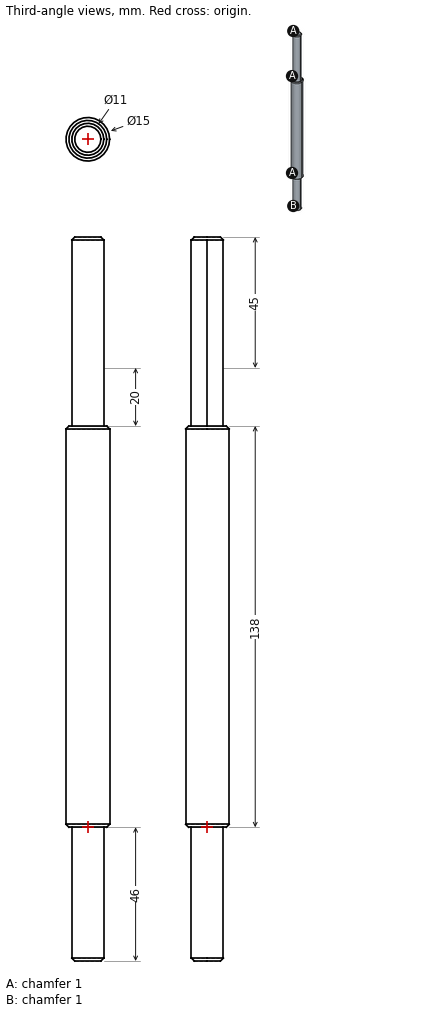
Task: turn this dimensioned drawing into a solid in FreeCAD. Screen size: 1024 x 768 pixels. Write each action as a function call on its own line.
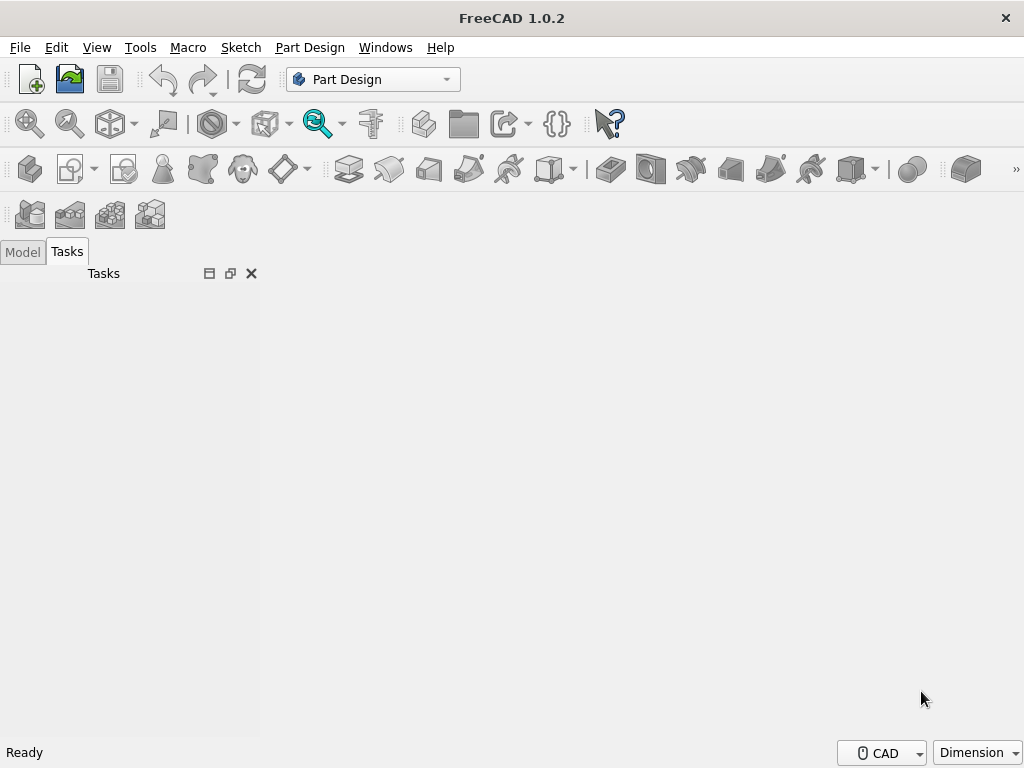
click(424, 170)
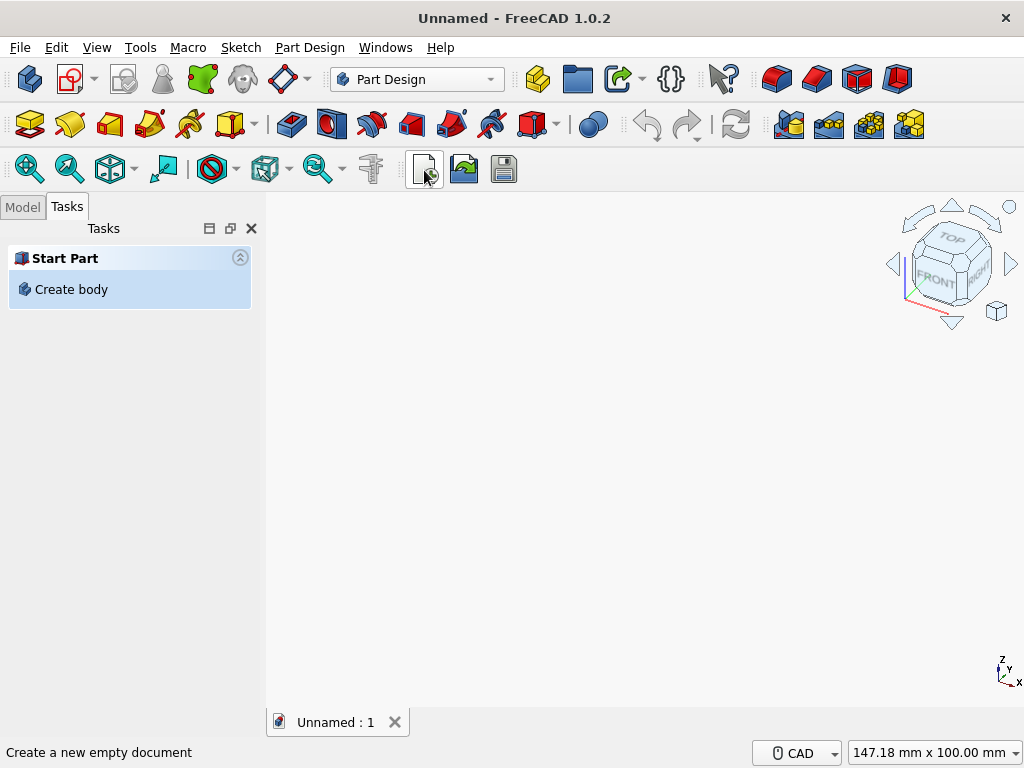
click(70, 80)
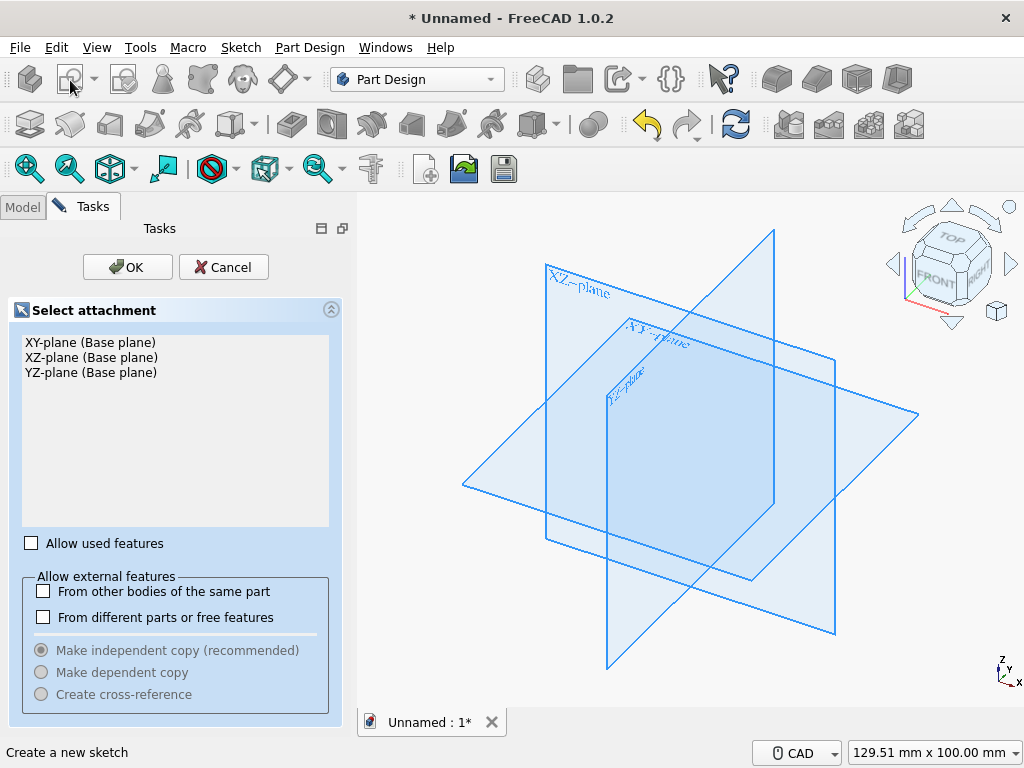
click(82, 342)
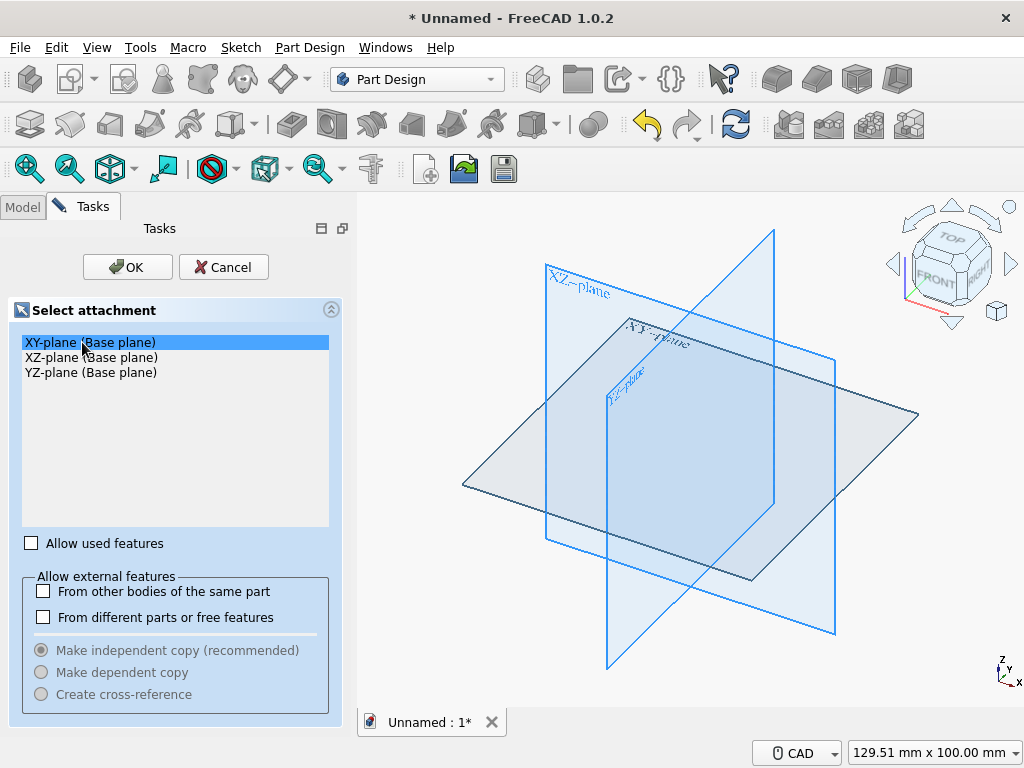
click(128, 267)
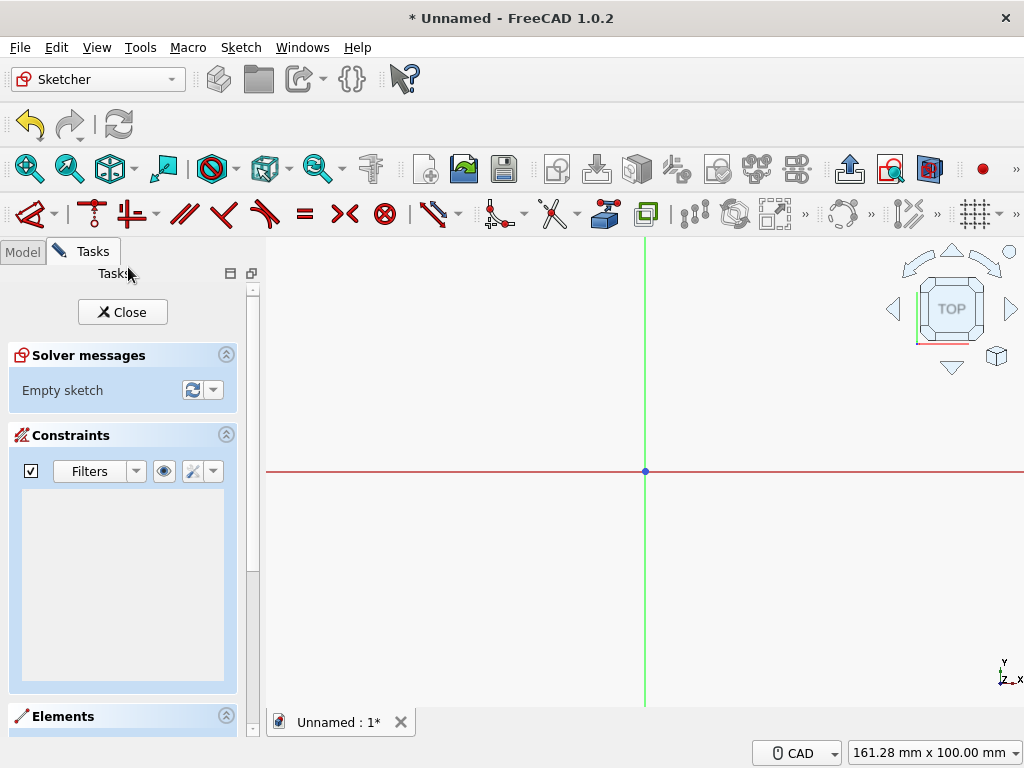
scroll(667, 472, up, 7)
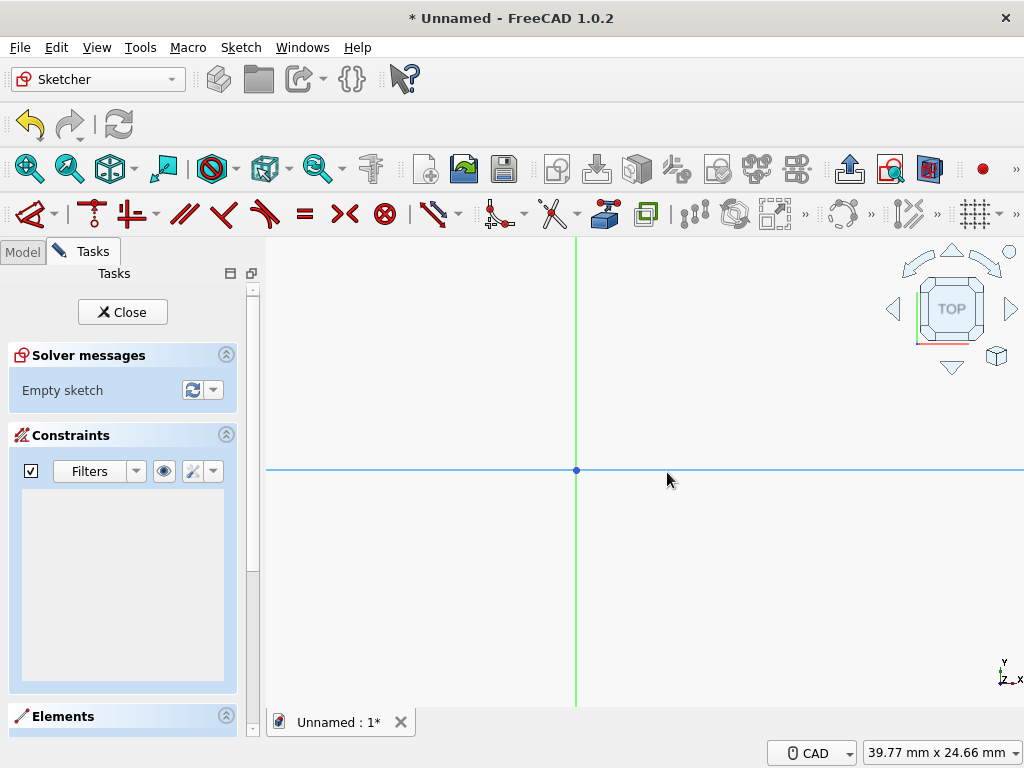
key(g)
key(c)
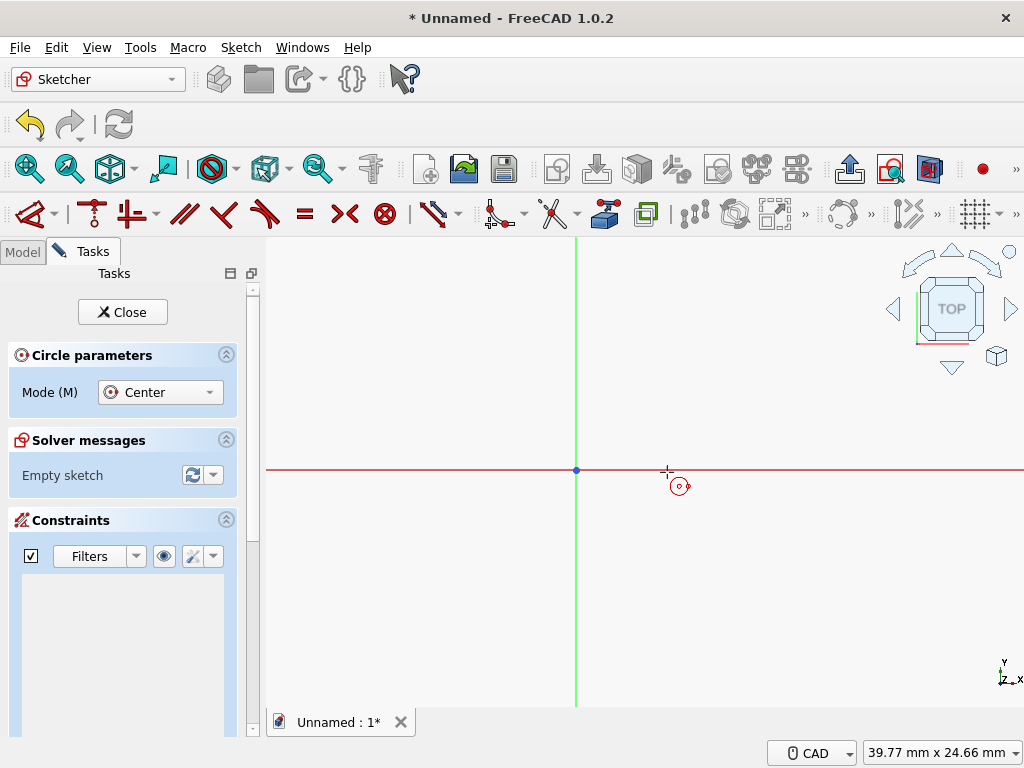
click(576, 470)
click(677, 369)
key(Escape)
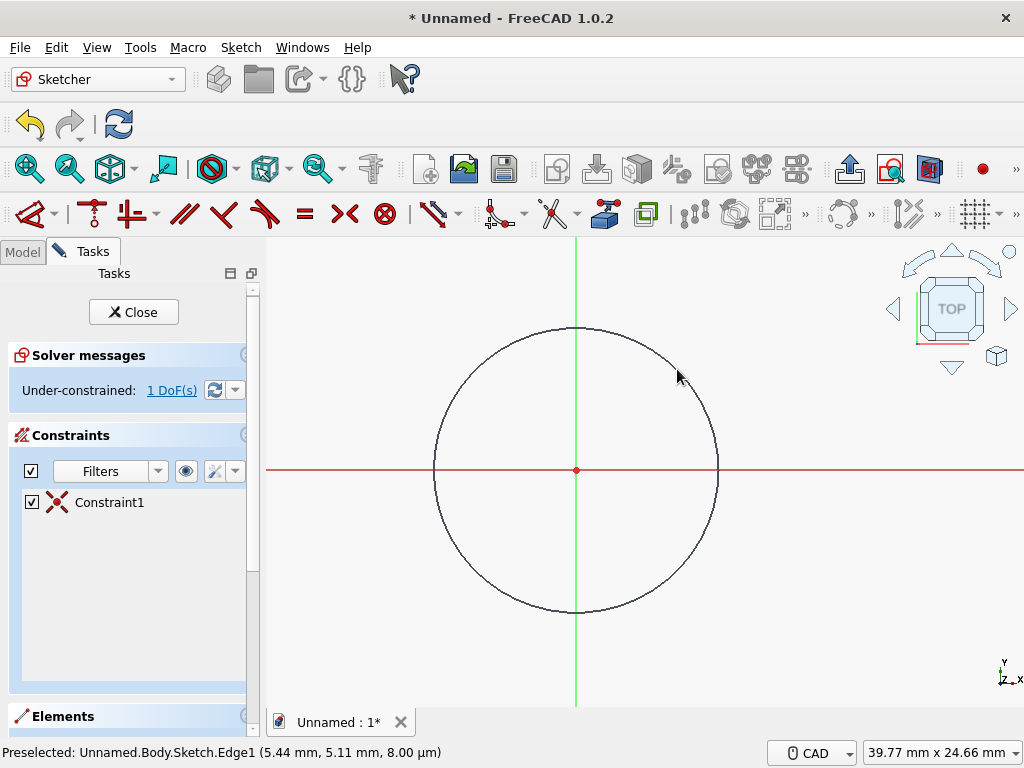
click(30, 214)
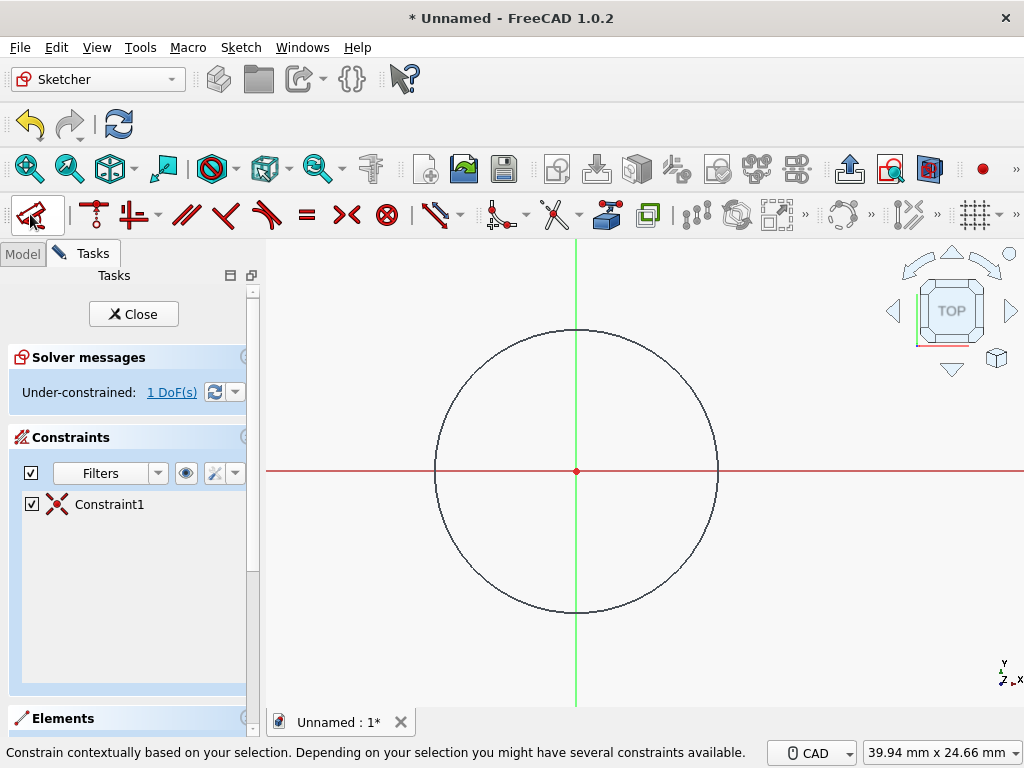
click(676, 371)
click(699, 348)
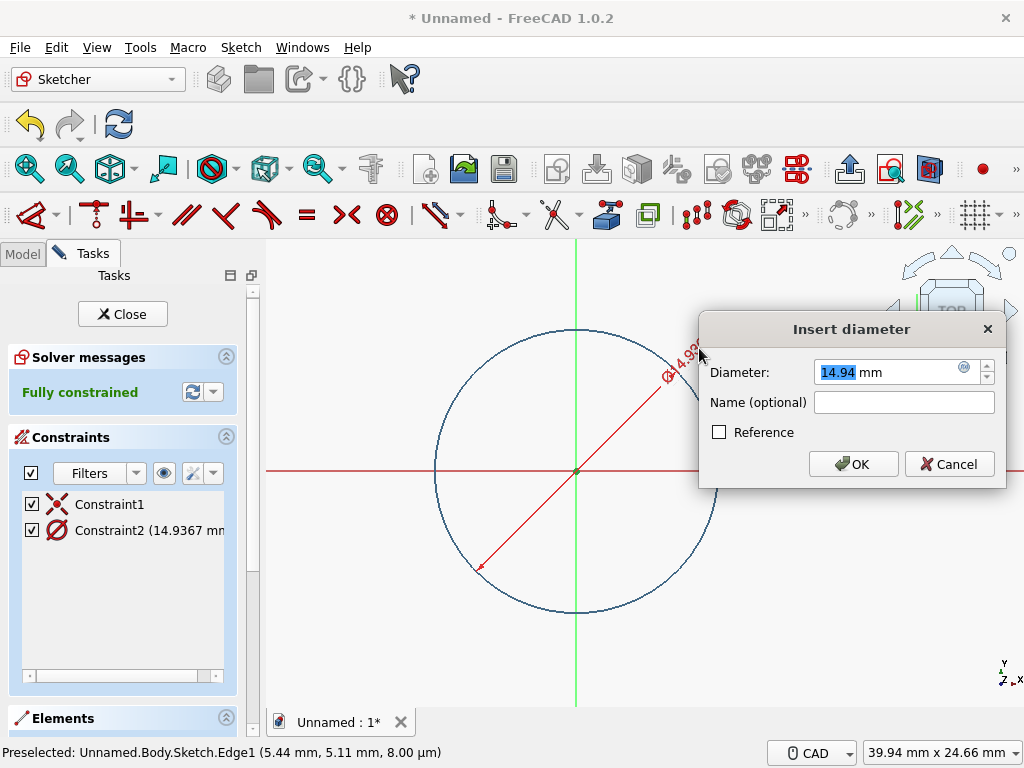
text(15)
key(Return)
key(Escape)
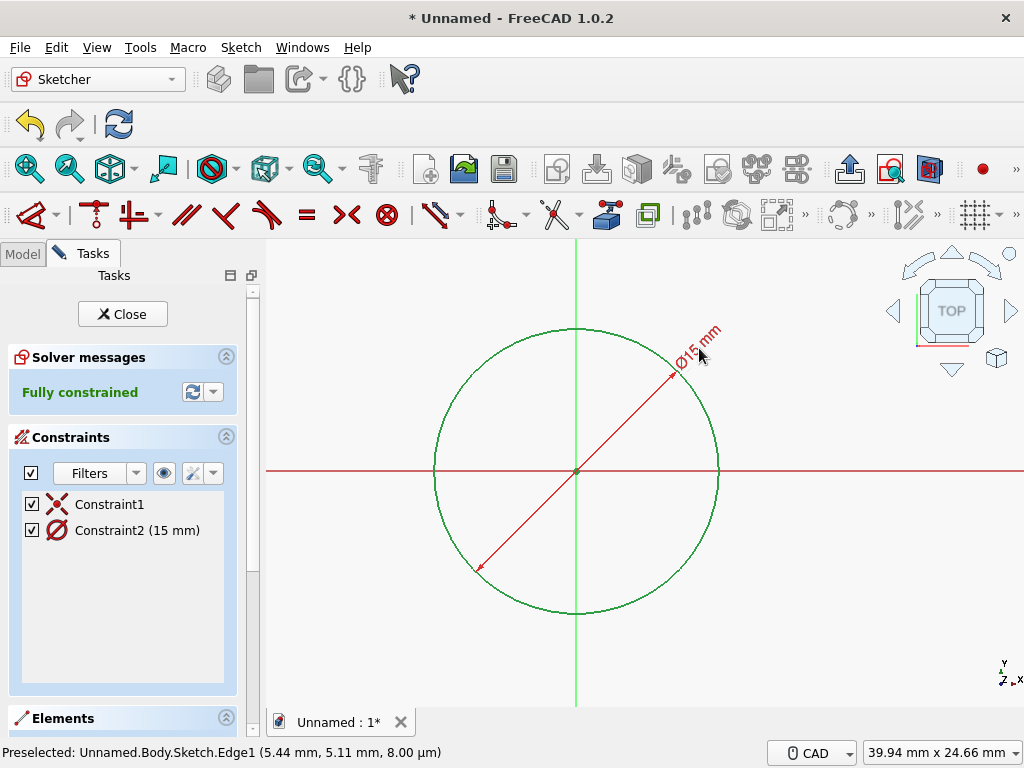
click(123, 314)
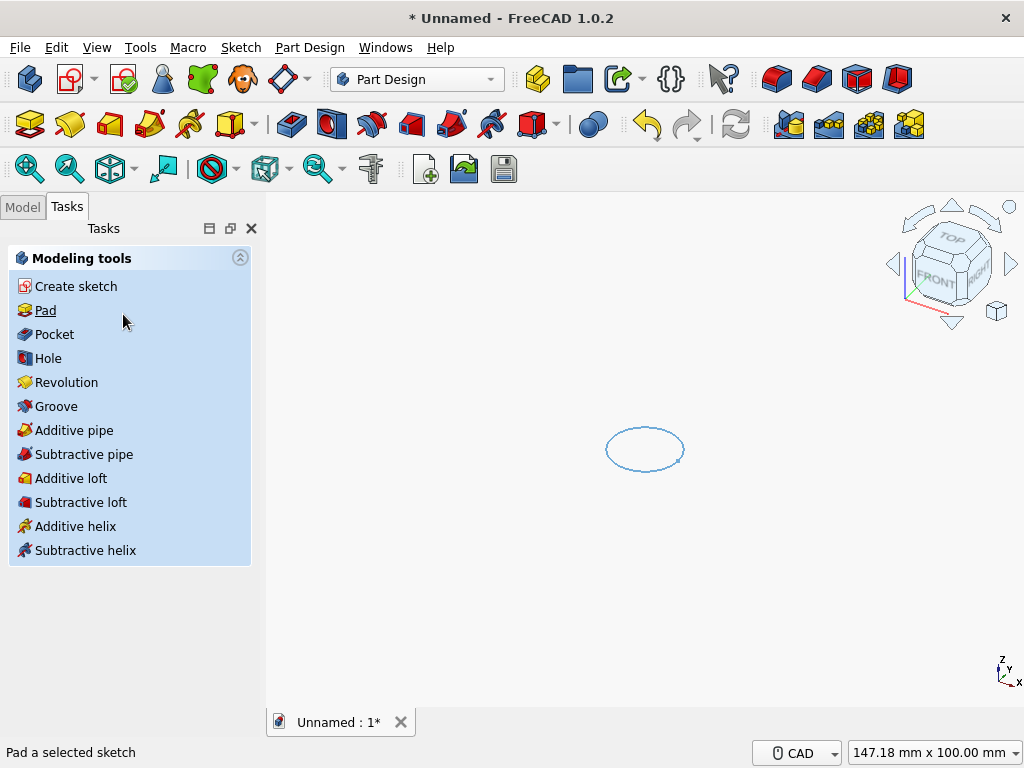
click(30, 124)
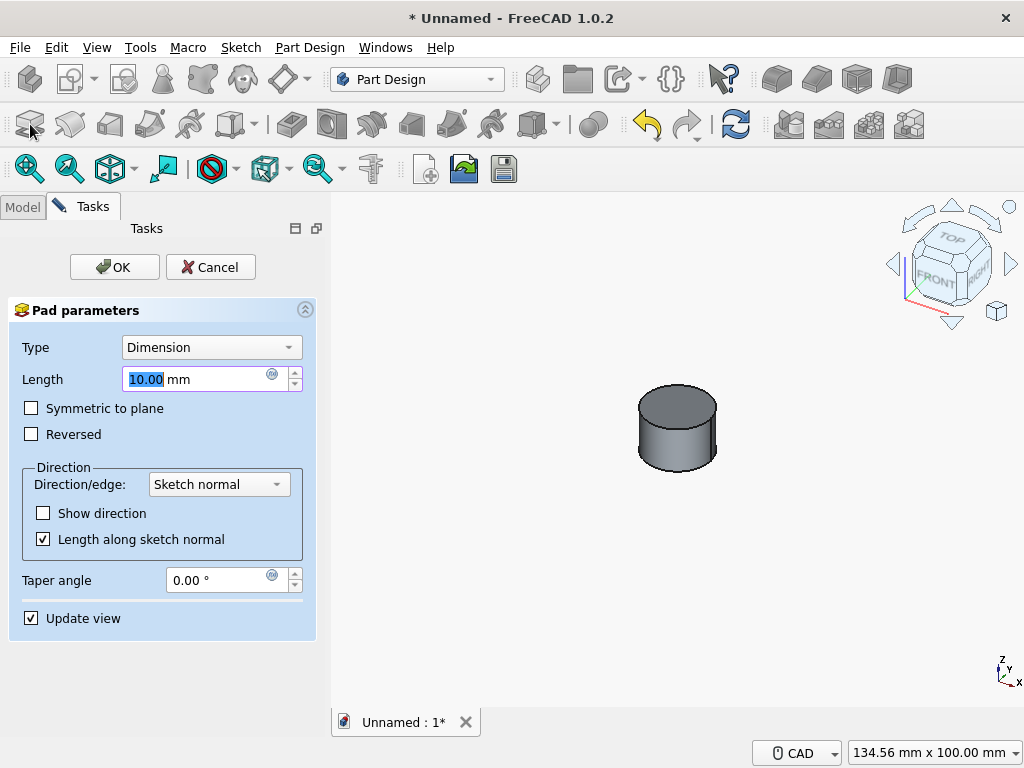
text(138)
key(Tab)